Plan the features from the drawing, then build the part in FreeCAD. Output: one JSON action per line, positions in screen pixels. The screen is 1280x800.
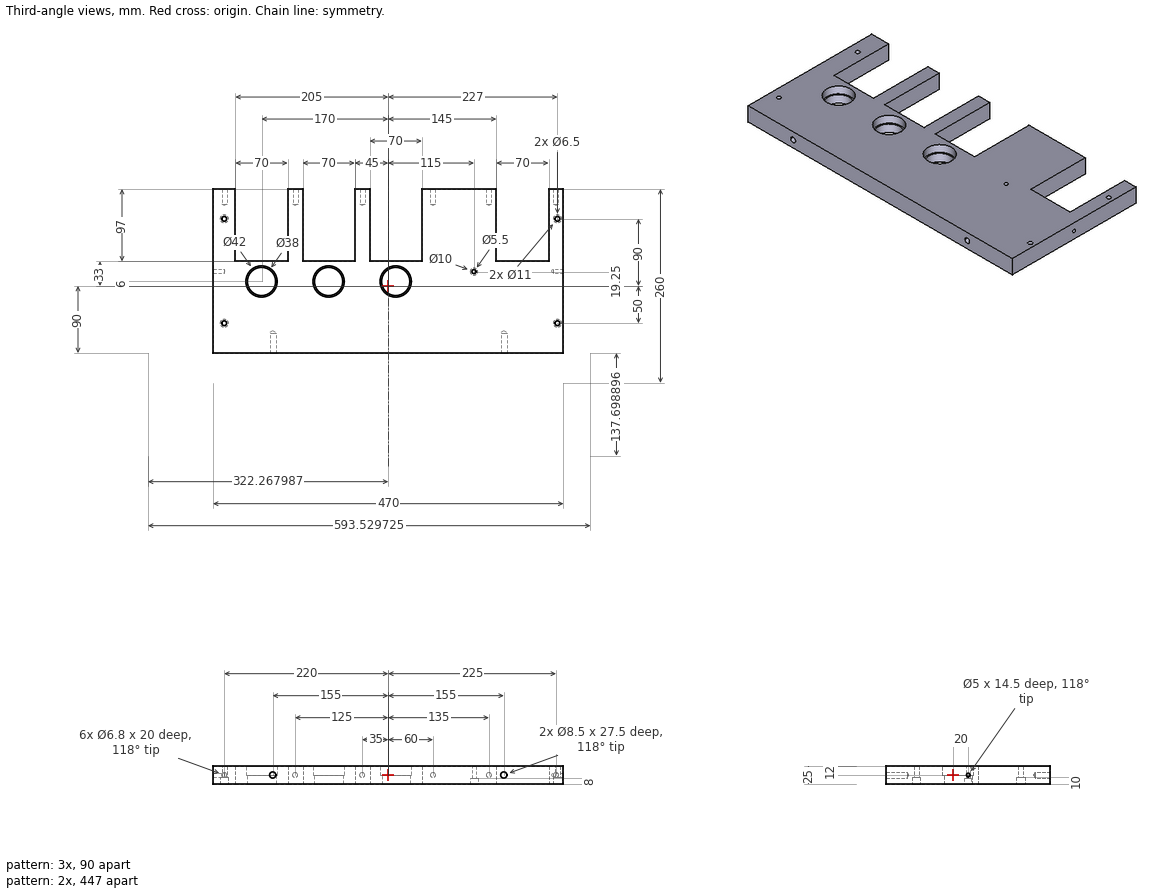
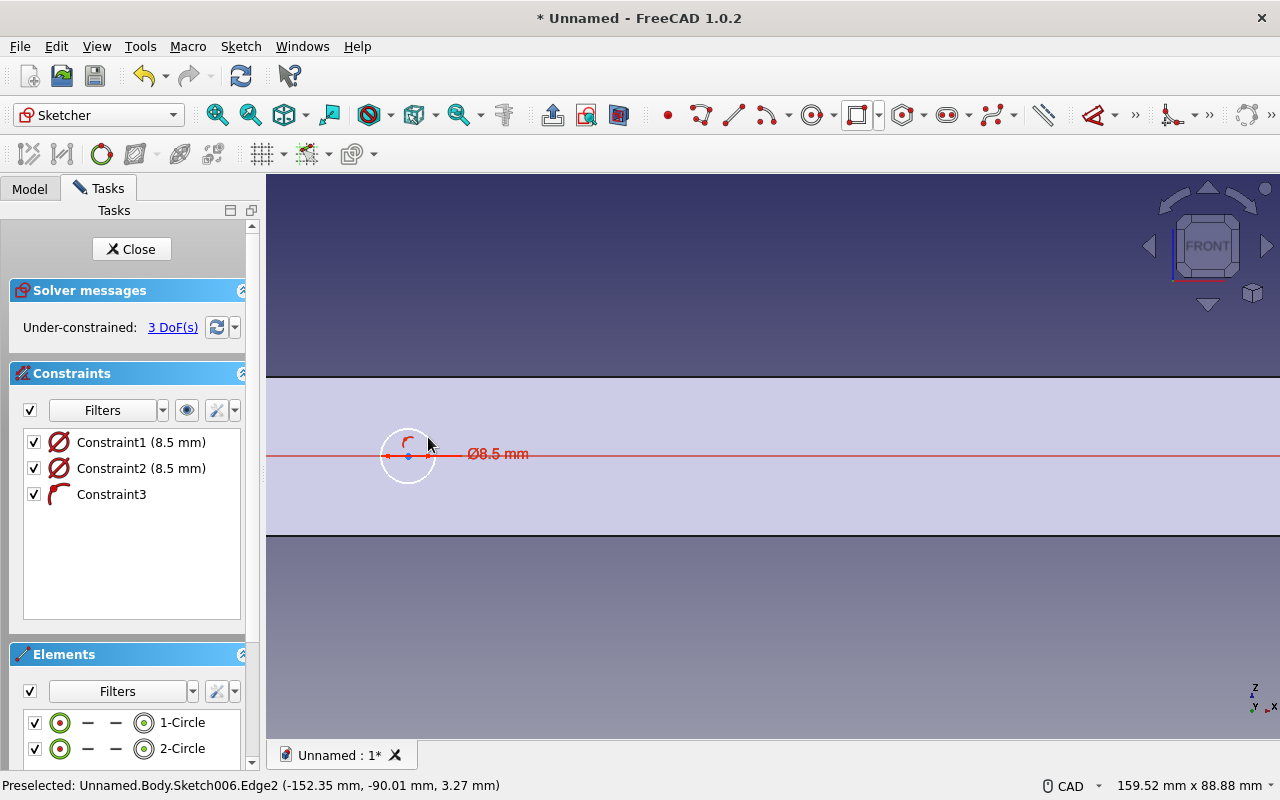
{"action": "scroll", "coordinate": [407, 457], "scroll_direction": "down", "scroll_amount": 6}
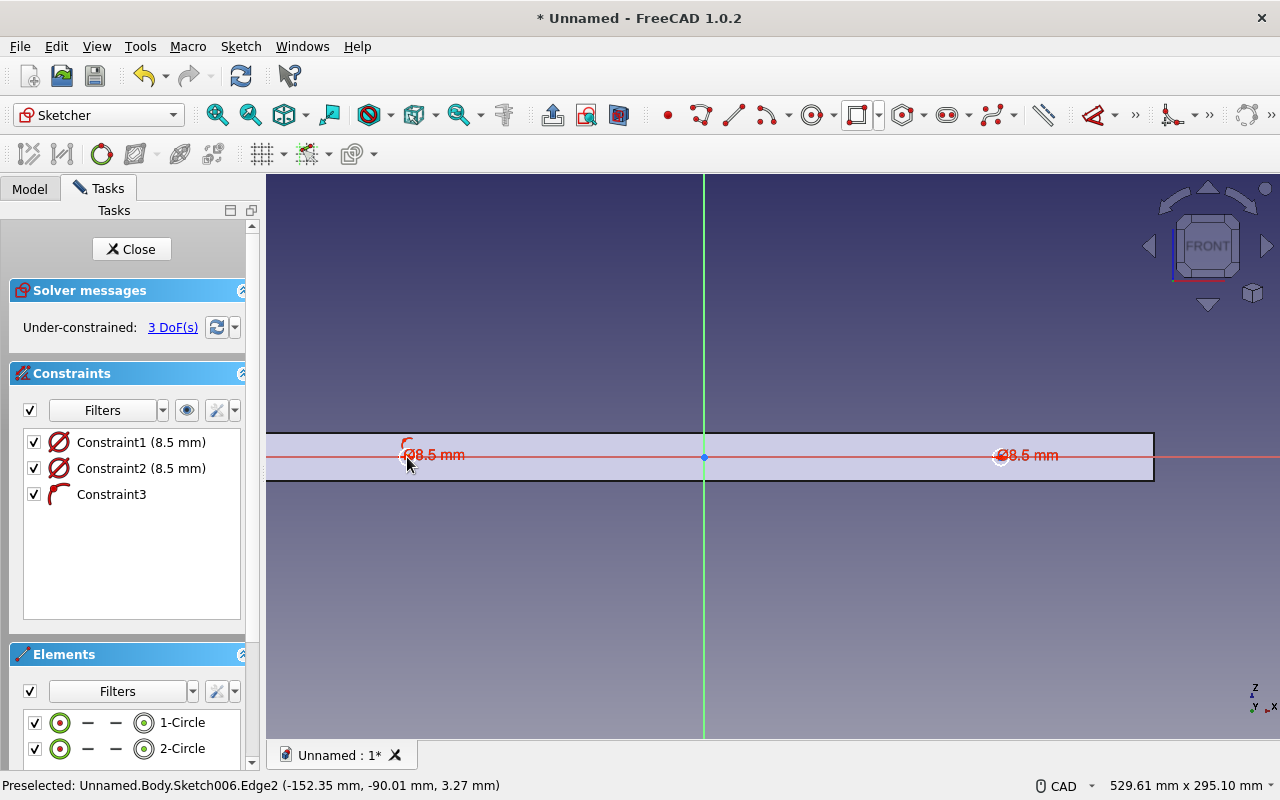
{"action": "left_click", "coordinate": [1001, 457]}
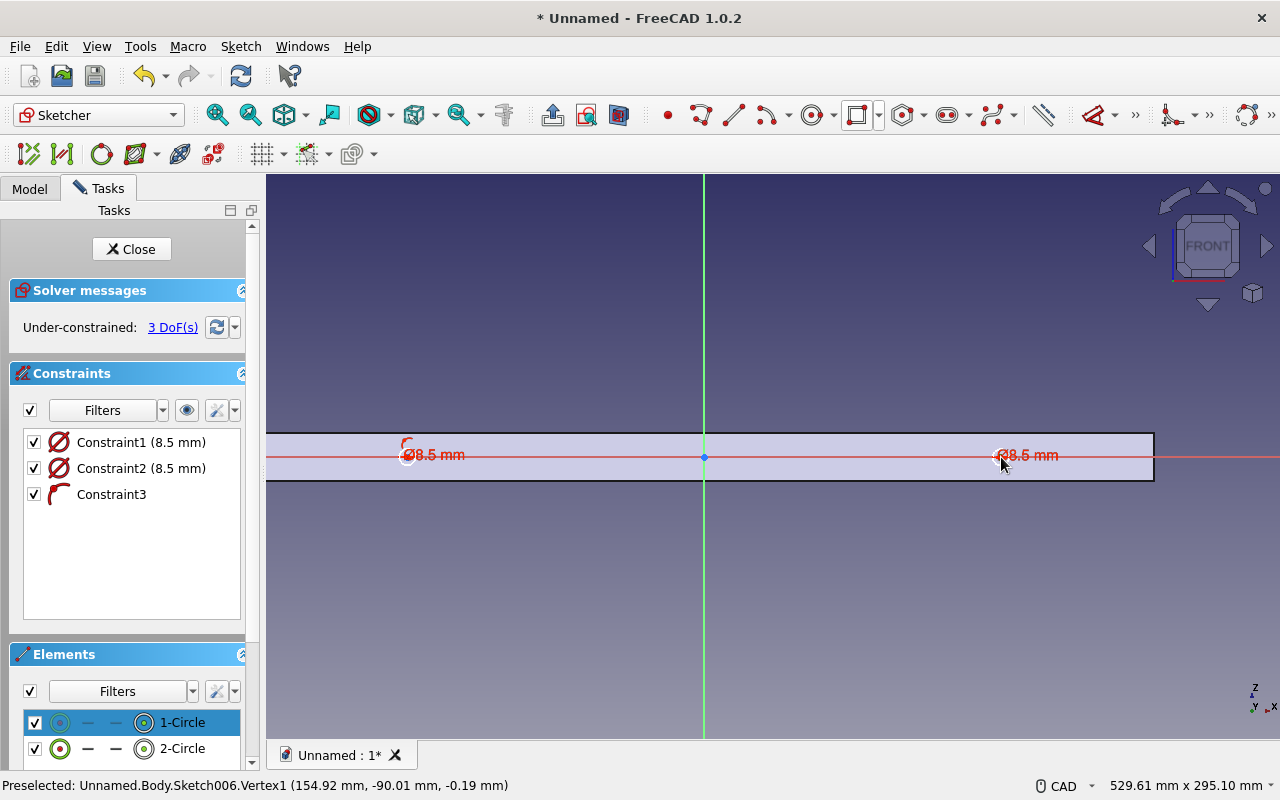
{"action": "left_click", "coordinate": [353, 457]}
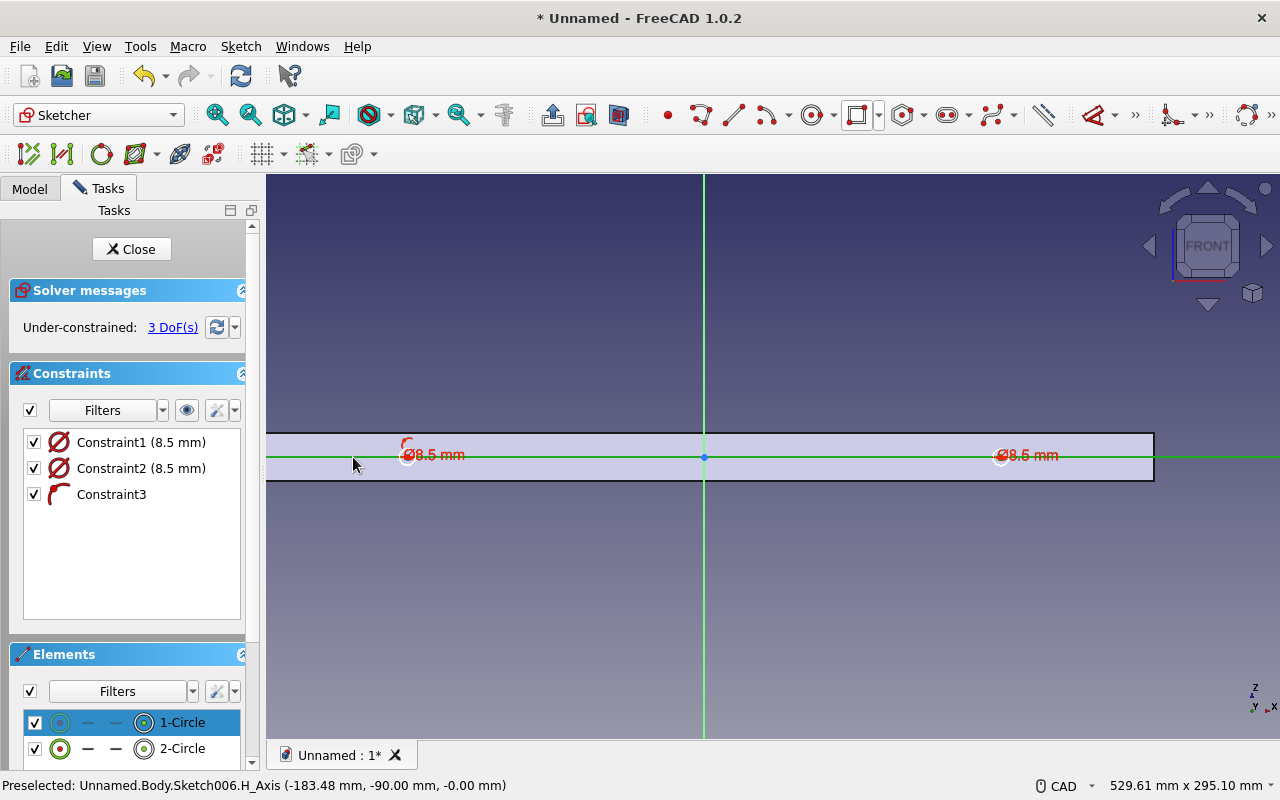
{"action": "key", "text": "c"}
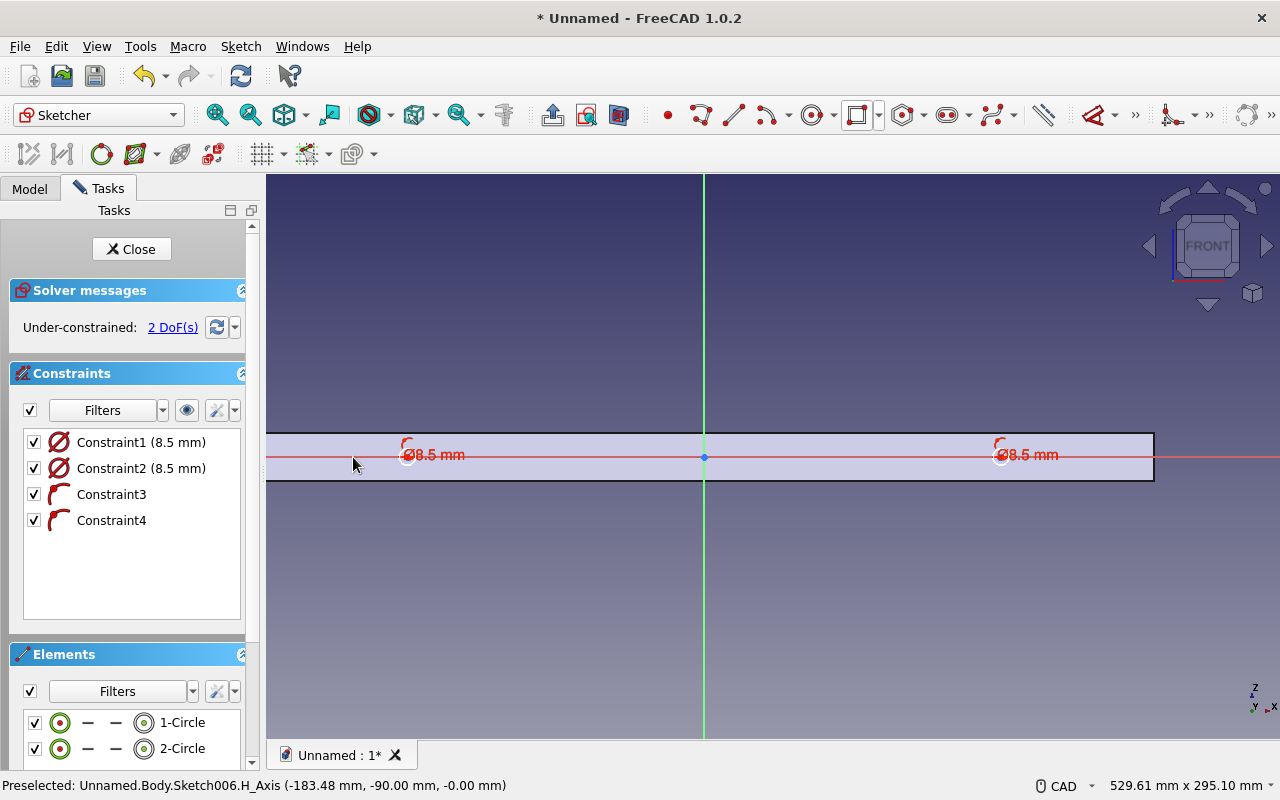
{"action": "left_click", "coordinate": [1092, 116]}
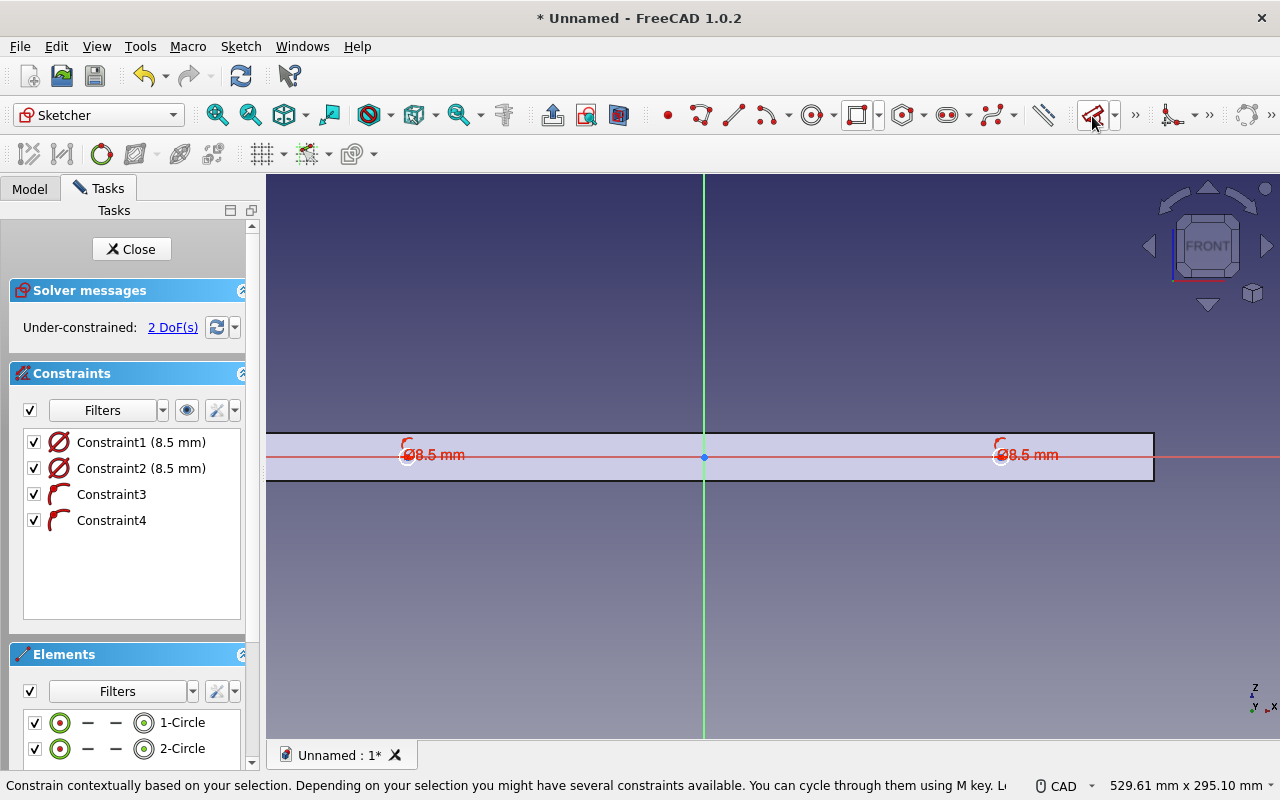
{"action": "left_click", "coordinate": [1001, 457]}
{"action": "left_click", "coordinate": [853, 491]}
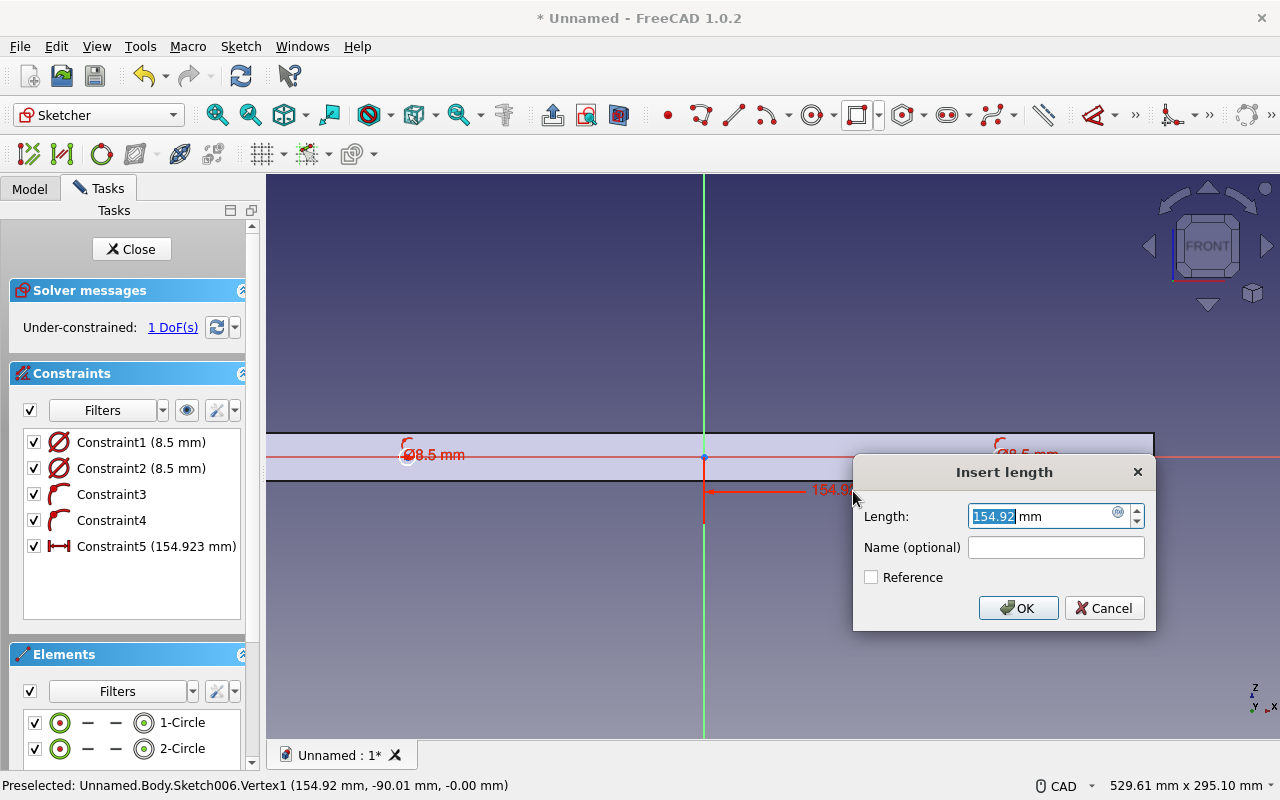
{"action": "type", "text": "155"}
{"action": "key", "text": "Return"}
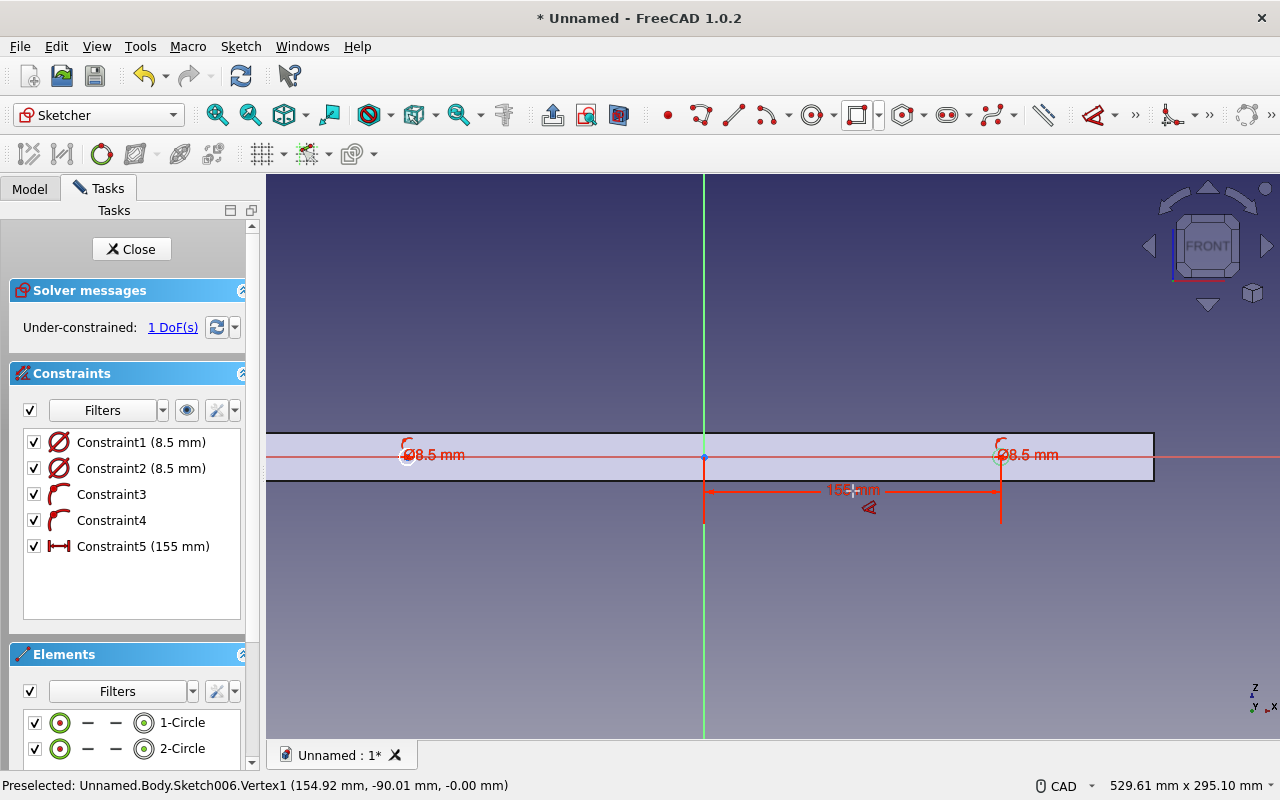
{"action": "left_click", "coordinate": [407, 457]}
{"action": "left_click", "coordinate": [556, 491]}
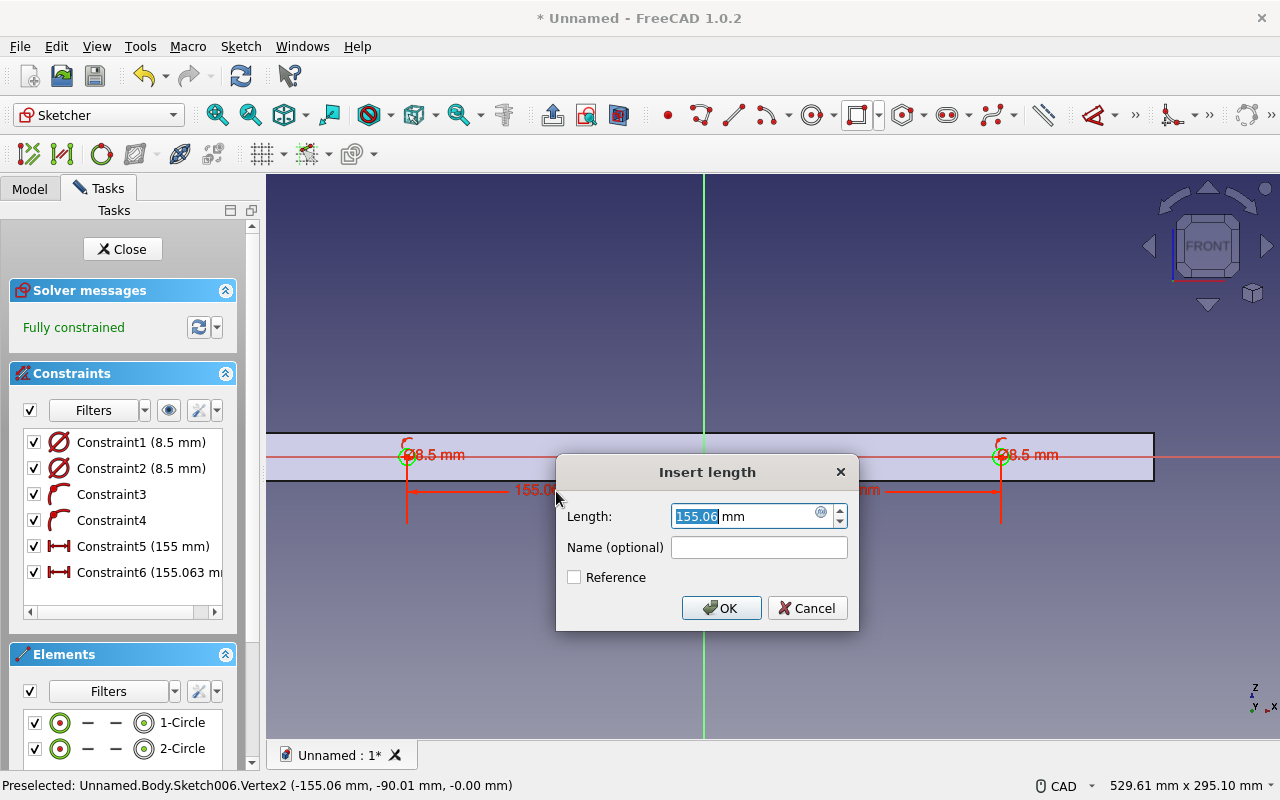
{"action": "type", "text": "155"}
{"action": "key", "text": "Return"}
{"action": "key", "text": "Escape"}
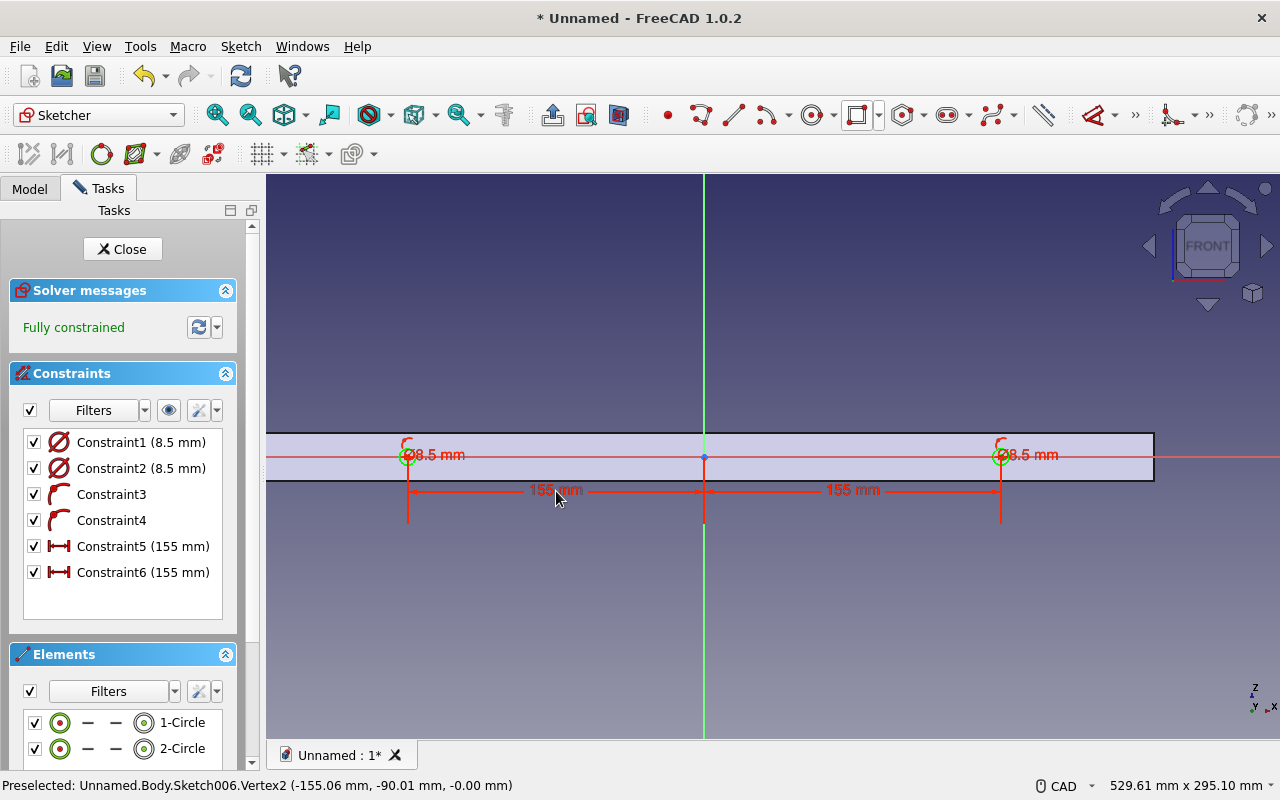
{"action": "left_click", "coordinate": [123, 249]}